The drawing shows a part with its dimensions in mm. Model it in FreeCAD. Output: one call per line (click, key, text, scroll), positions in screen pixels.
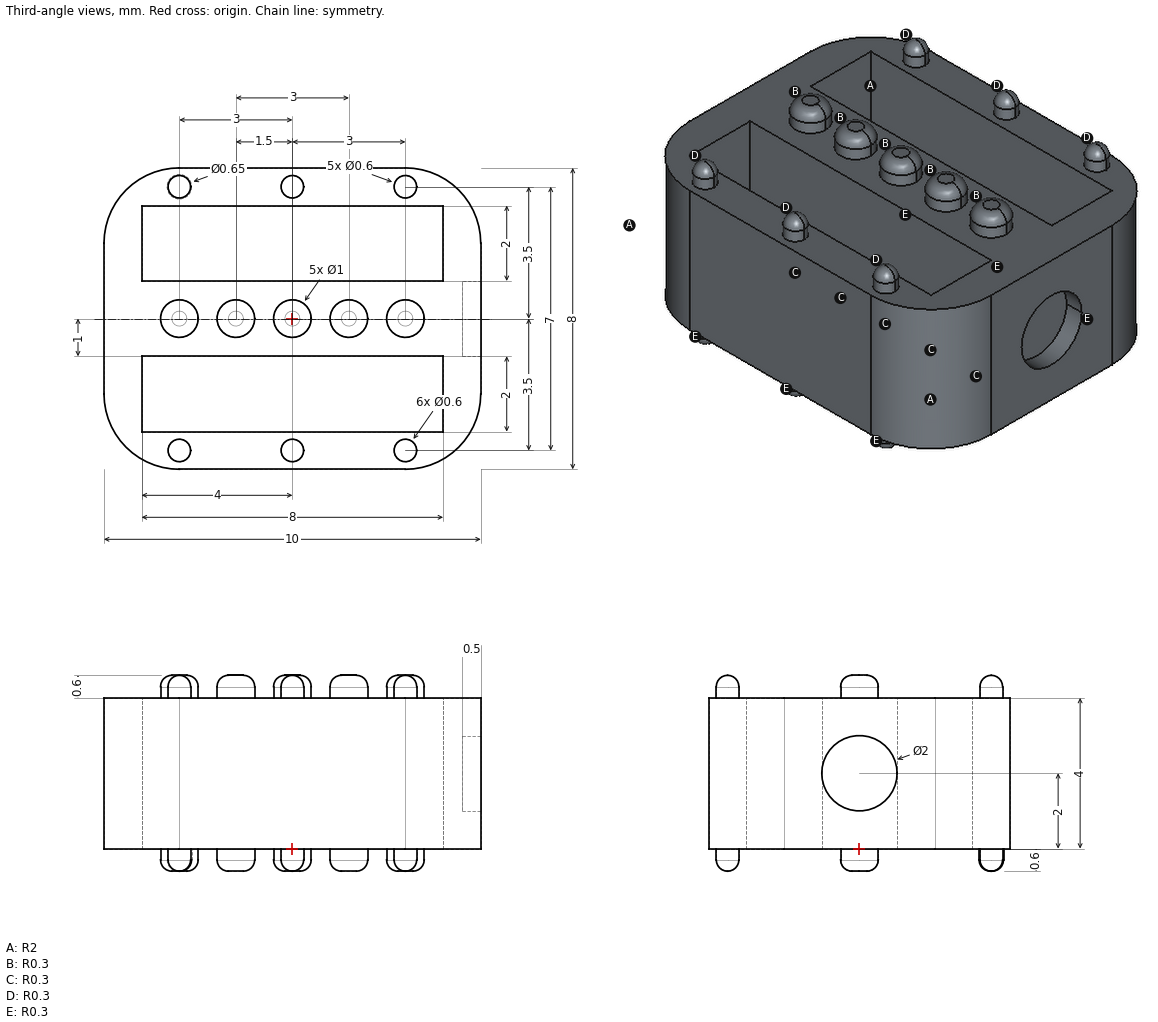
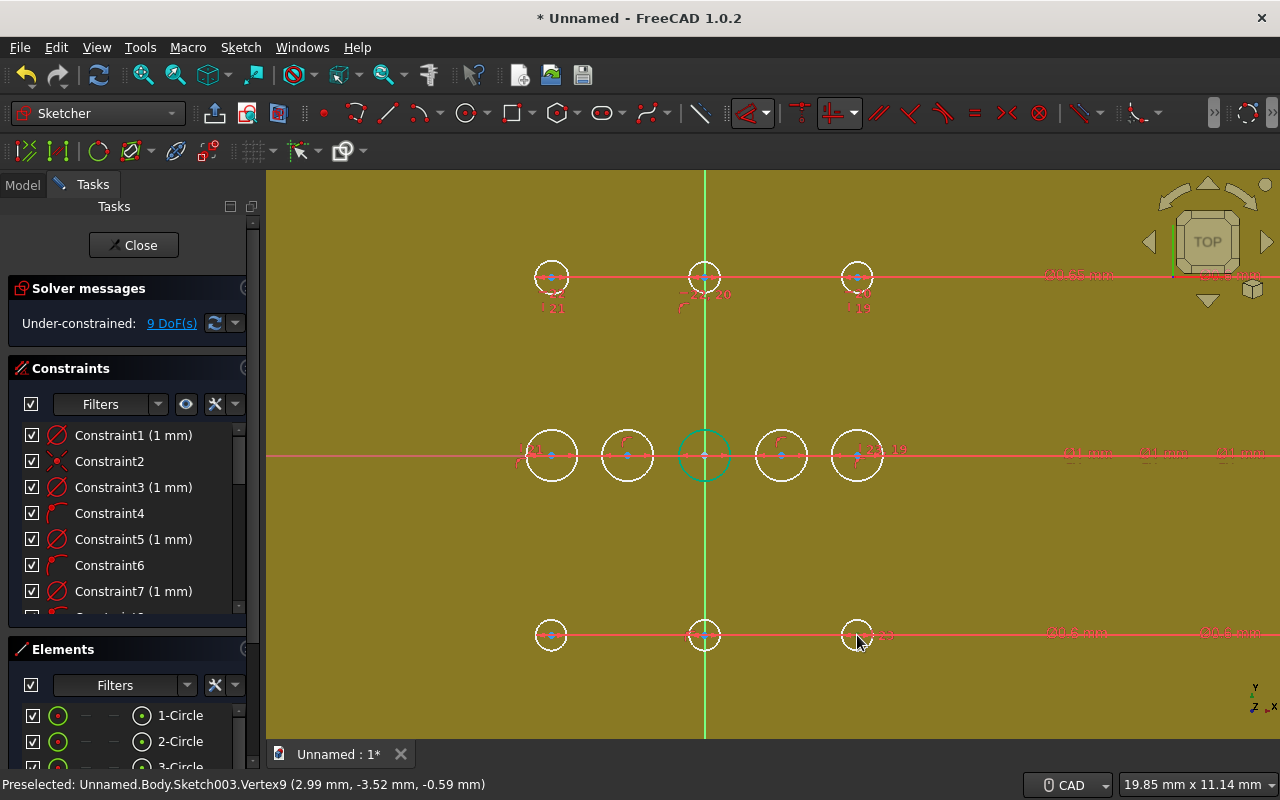
click(705, 635)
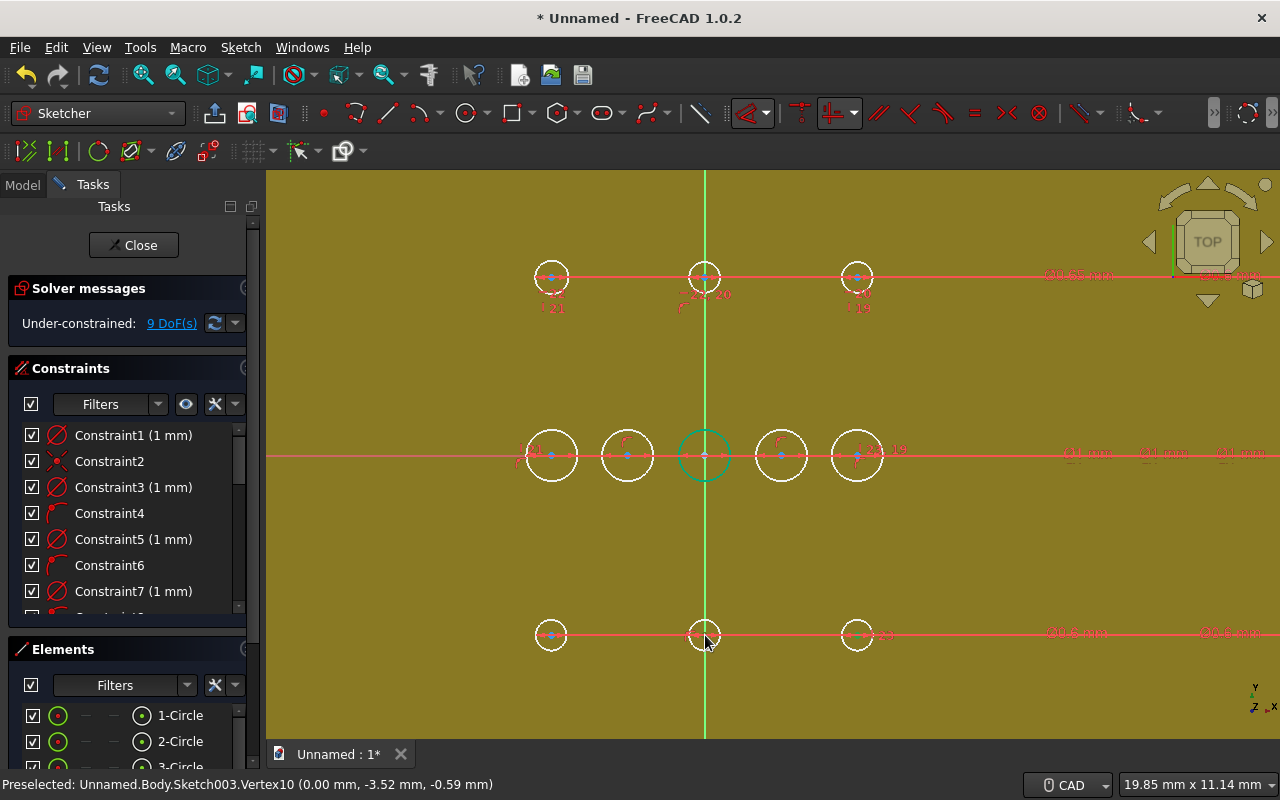
key(h)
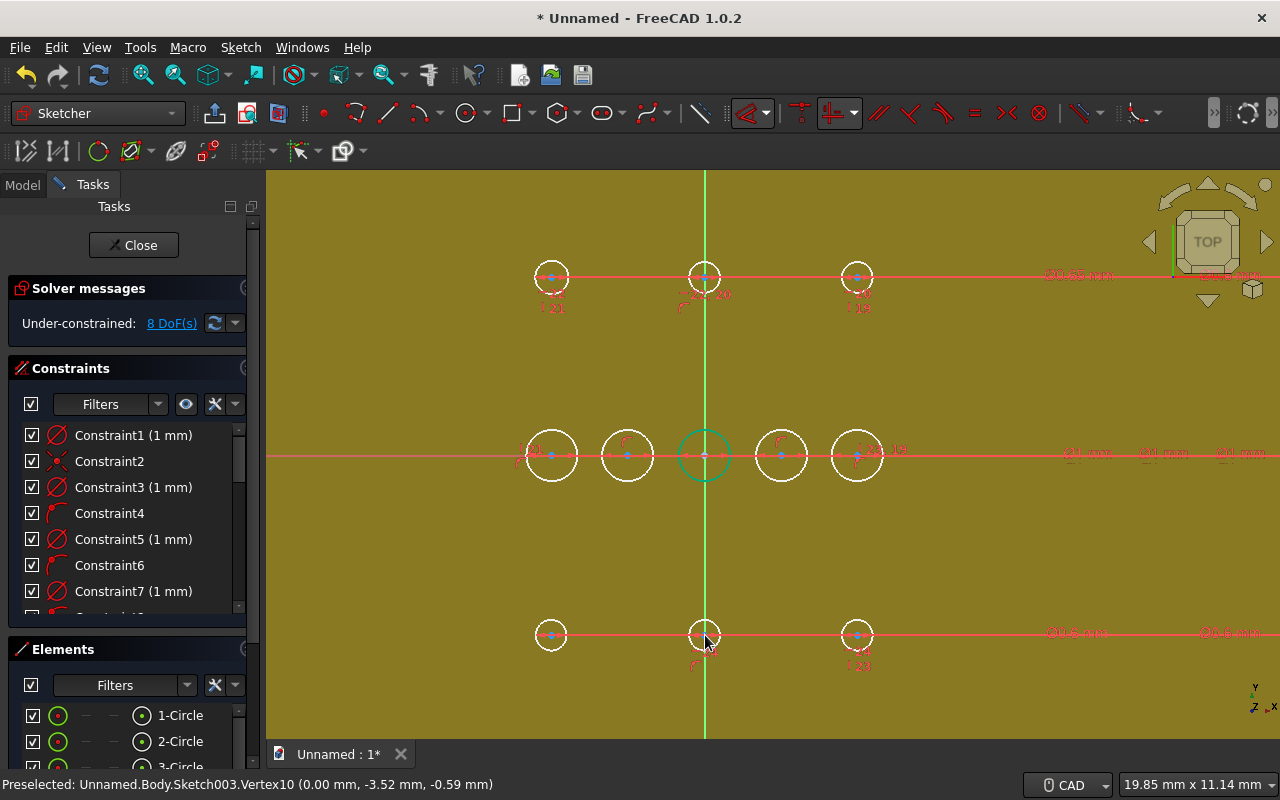
click(552, 456)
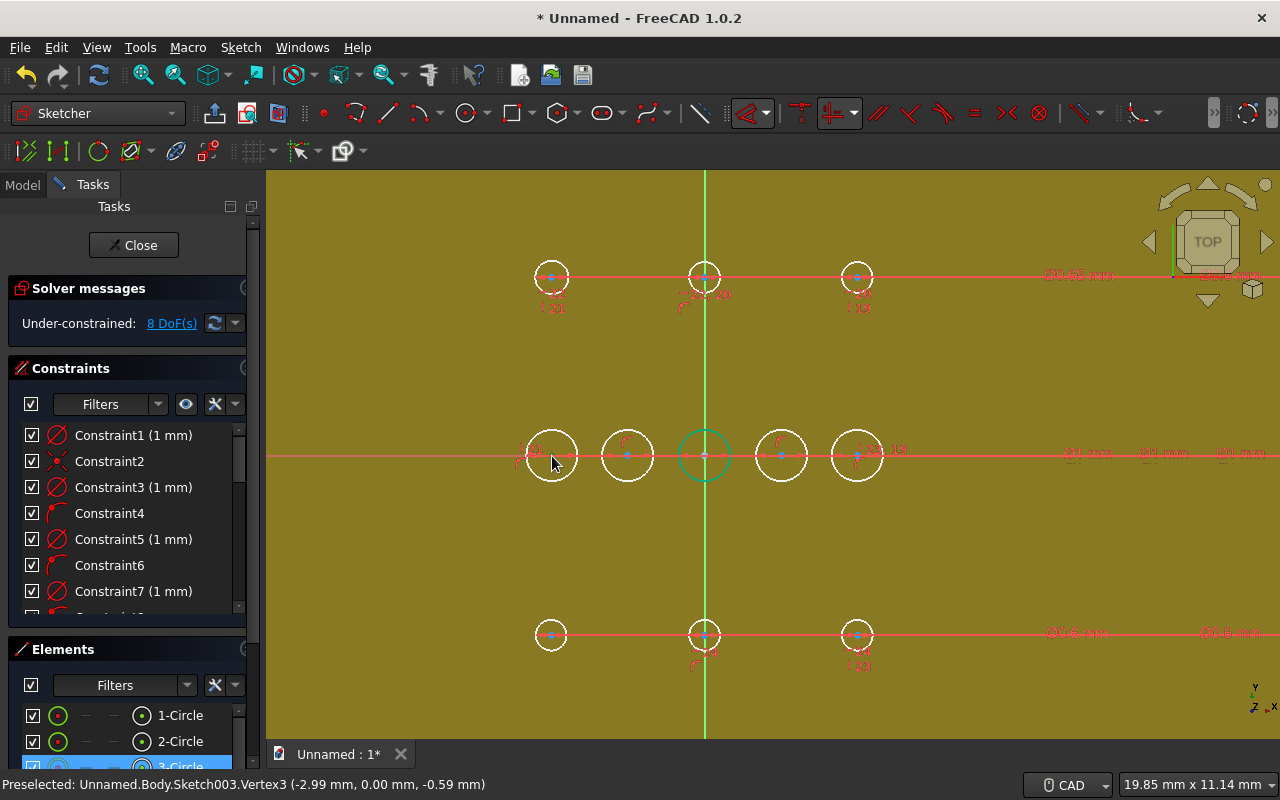
click(551, 635)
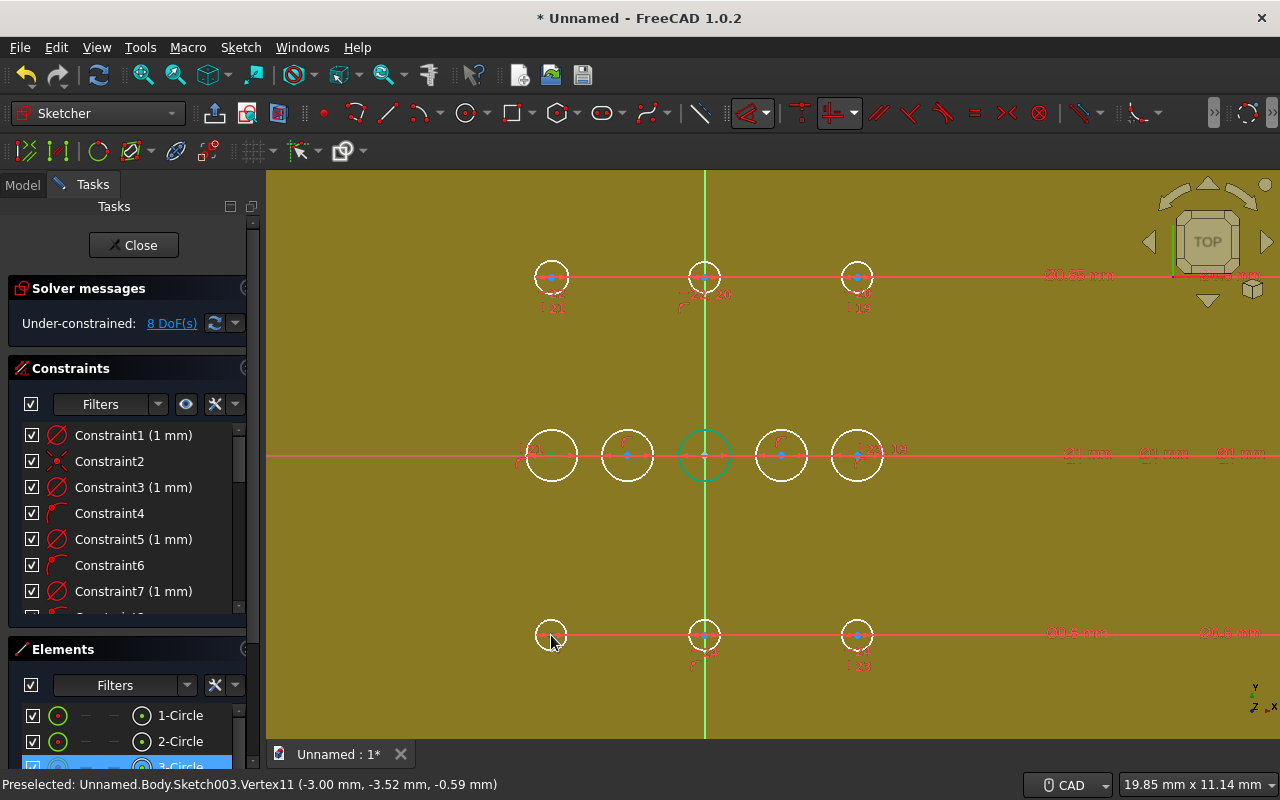
click(856, 114)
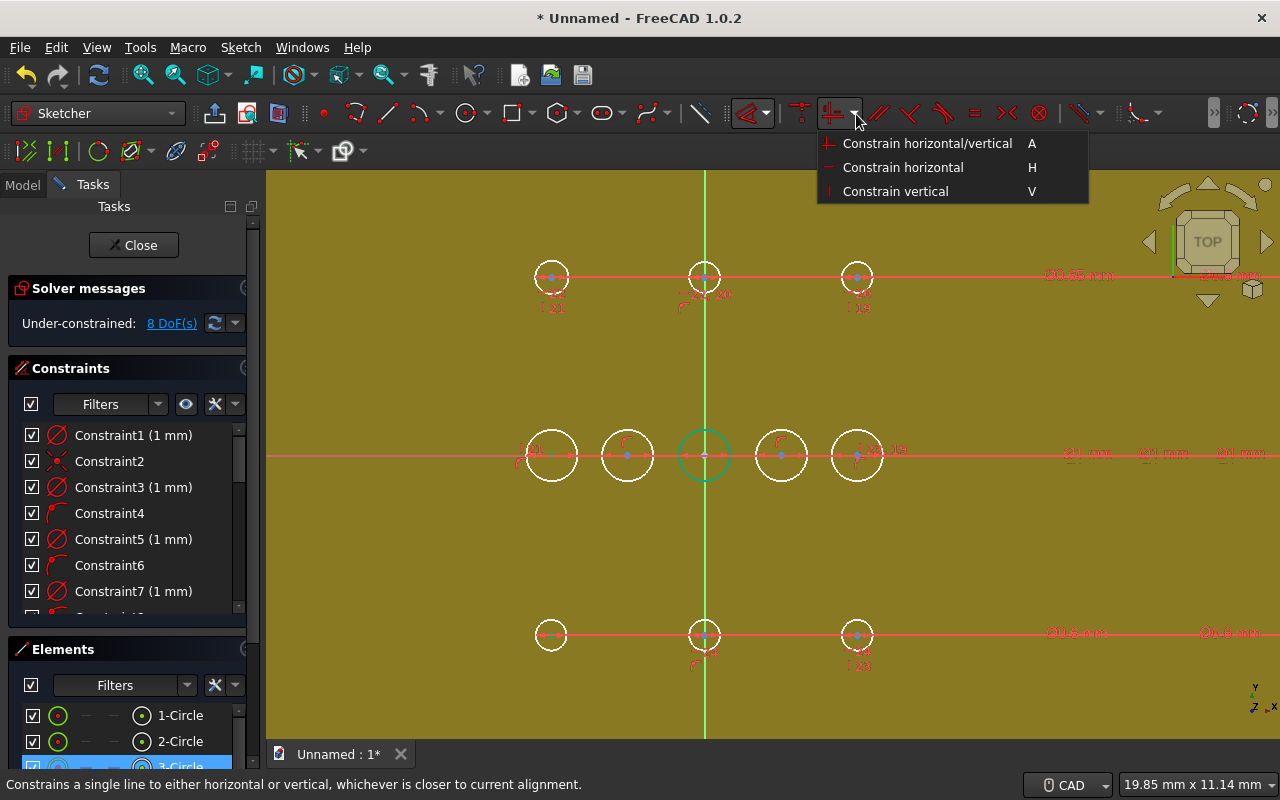
click(953, 191)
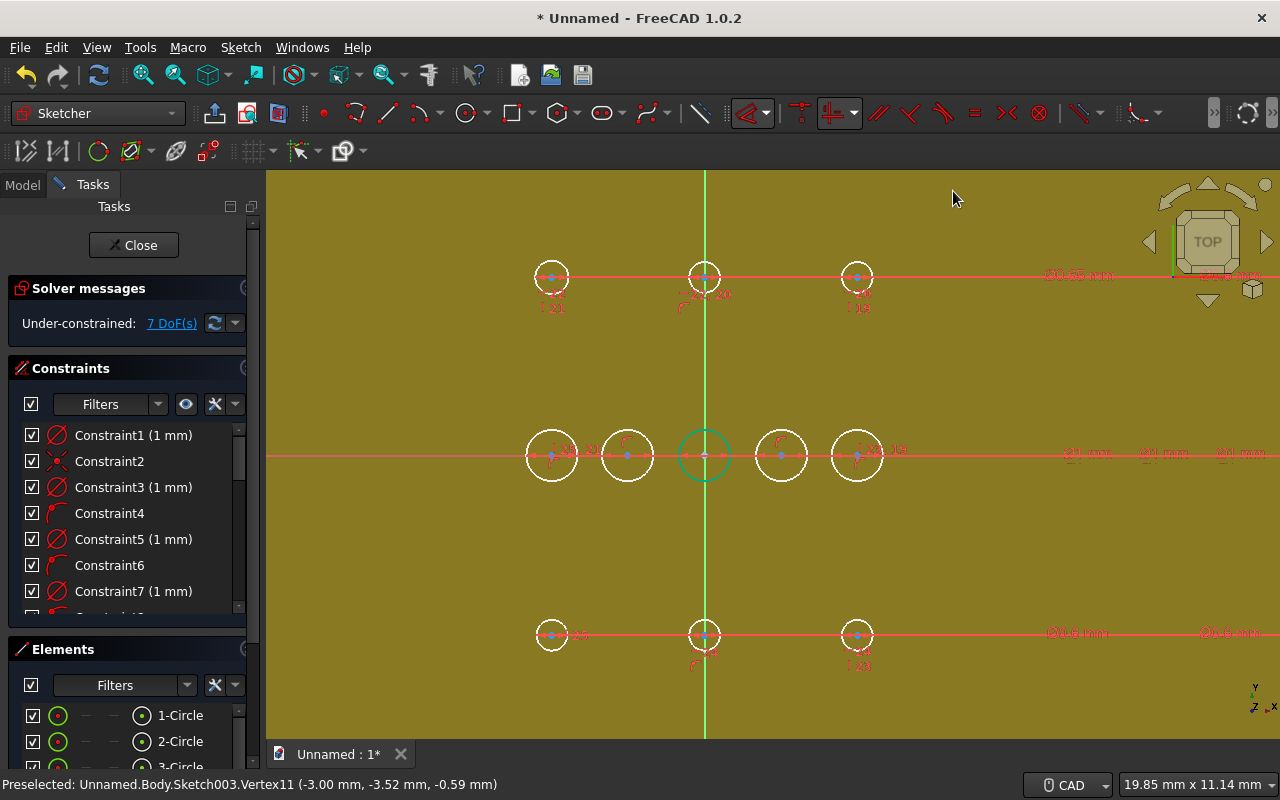
click(705, 635)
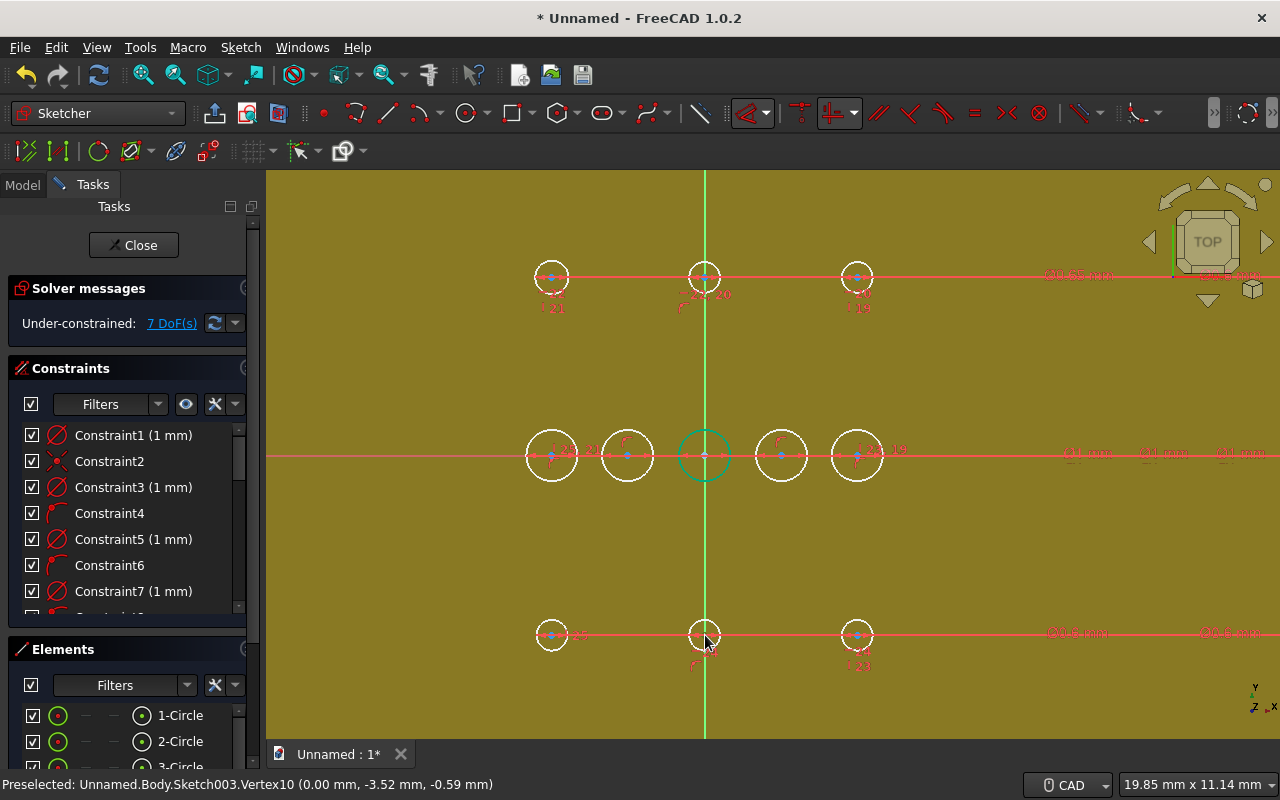
click(552, 635)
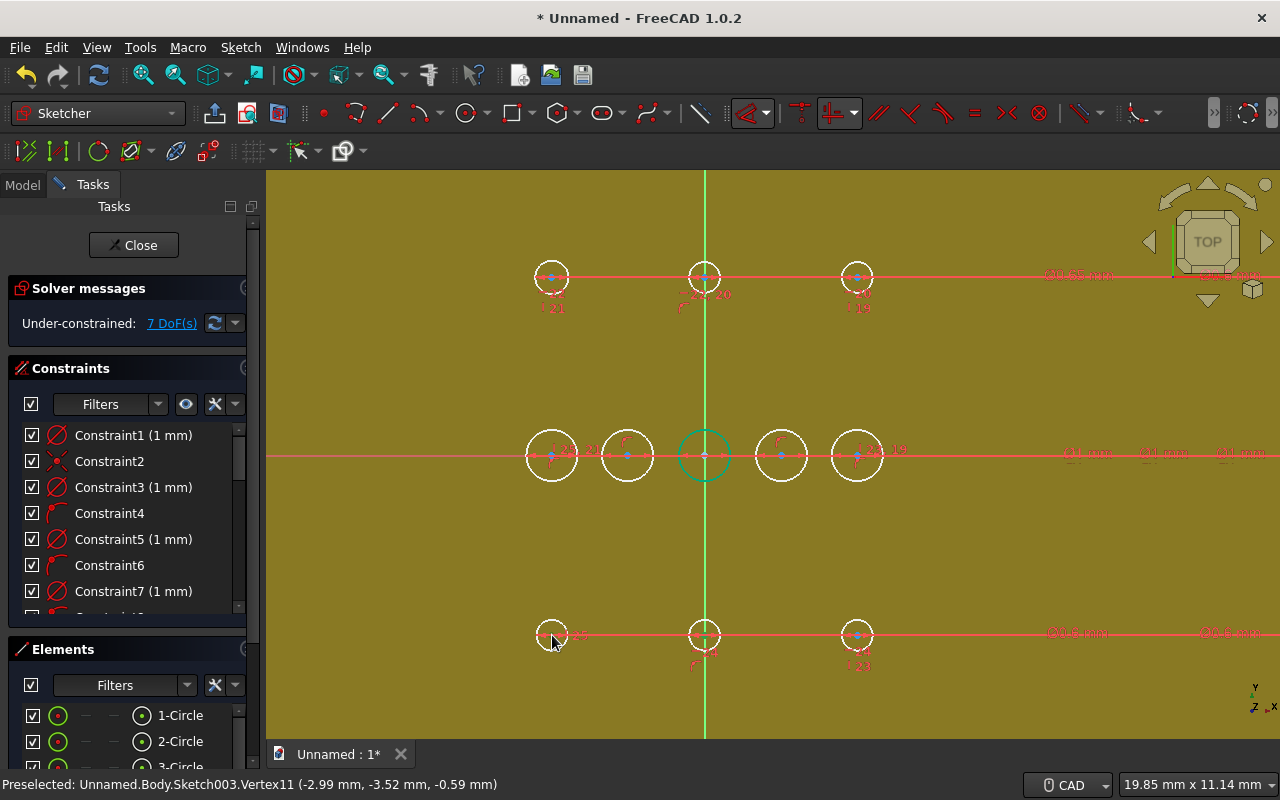
key(h)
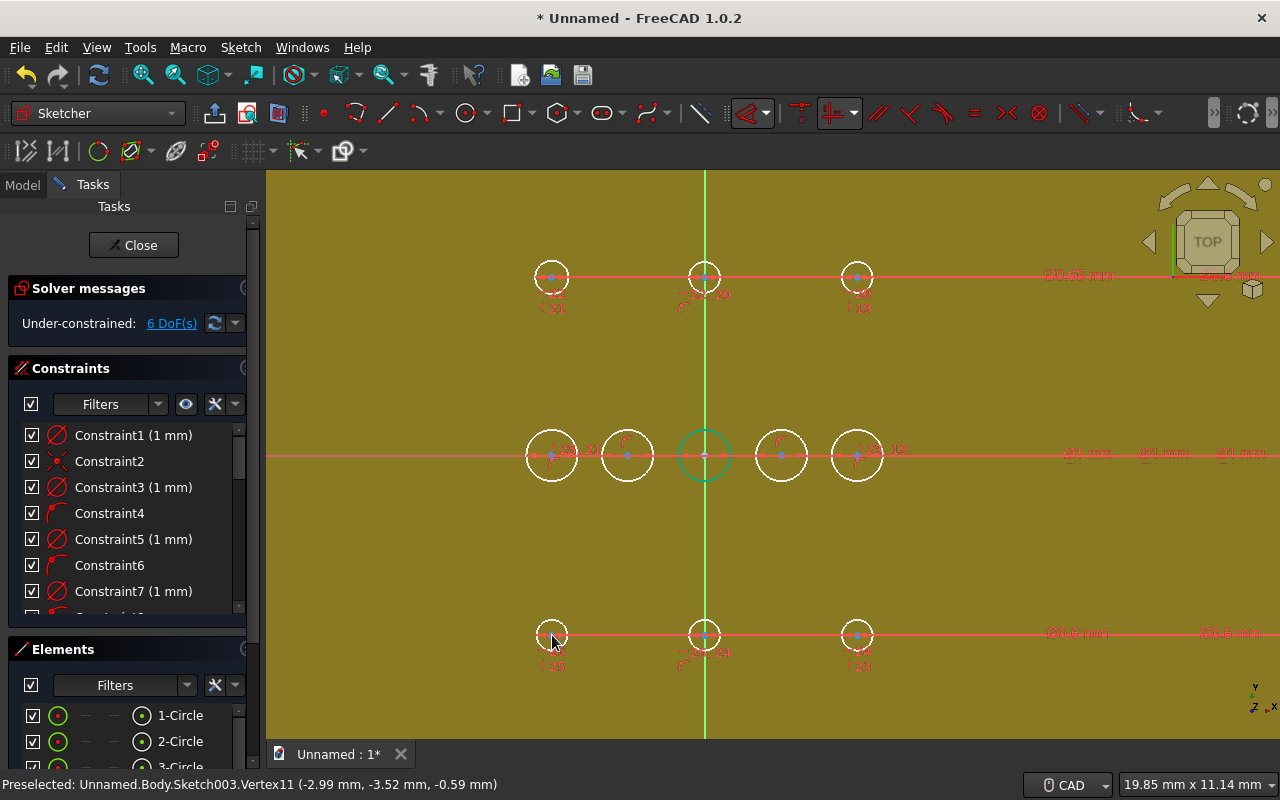
click(552, 456)